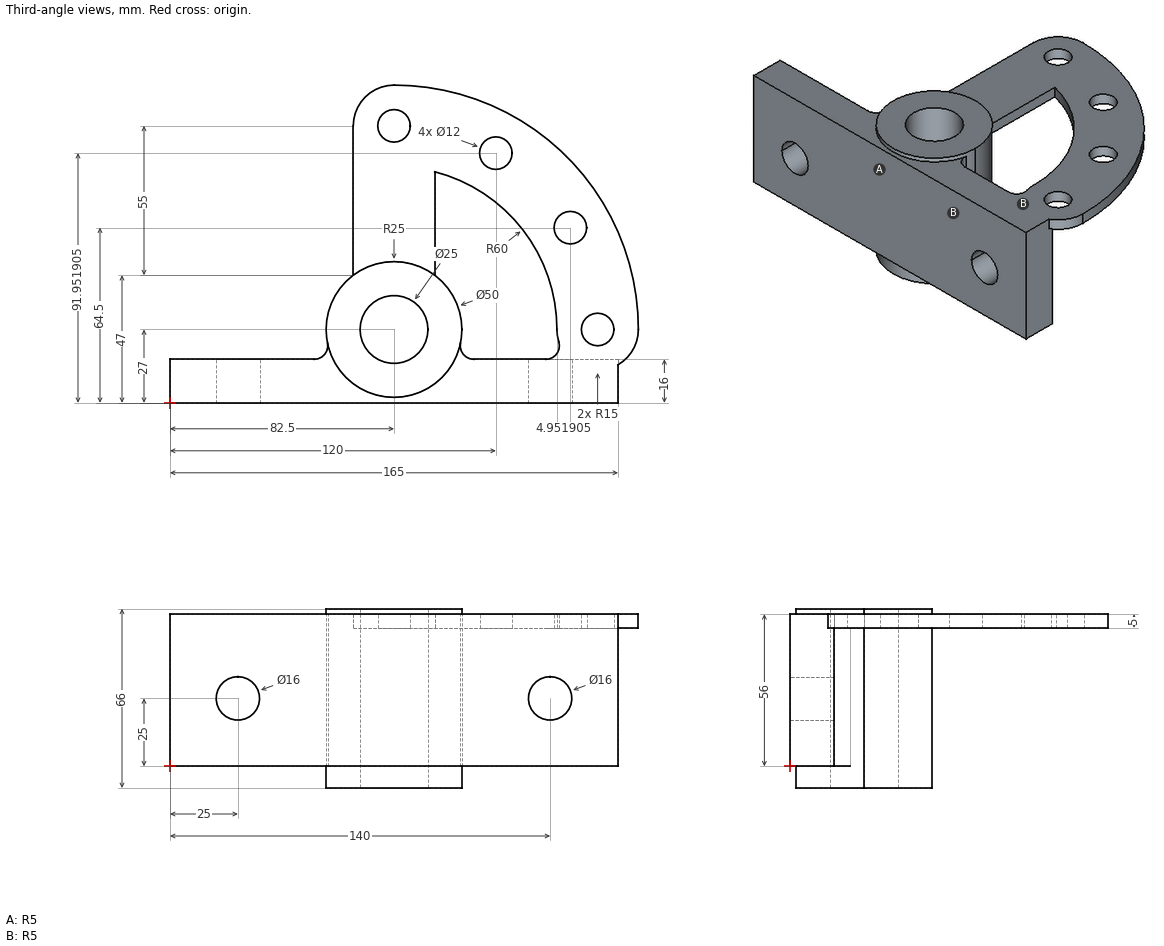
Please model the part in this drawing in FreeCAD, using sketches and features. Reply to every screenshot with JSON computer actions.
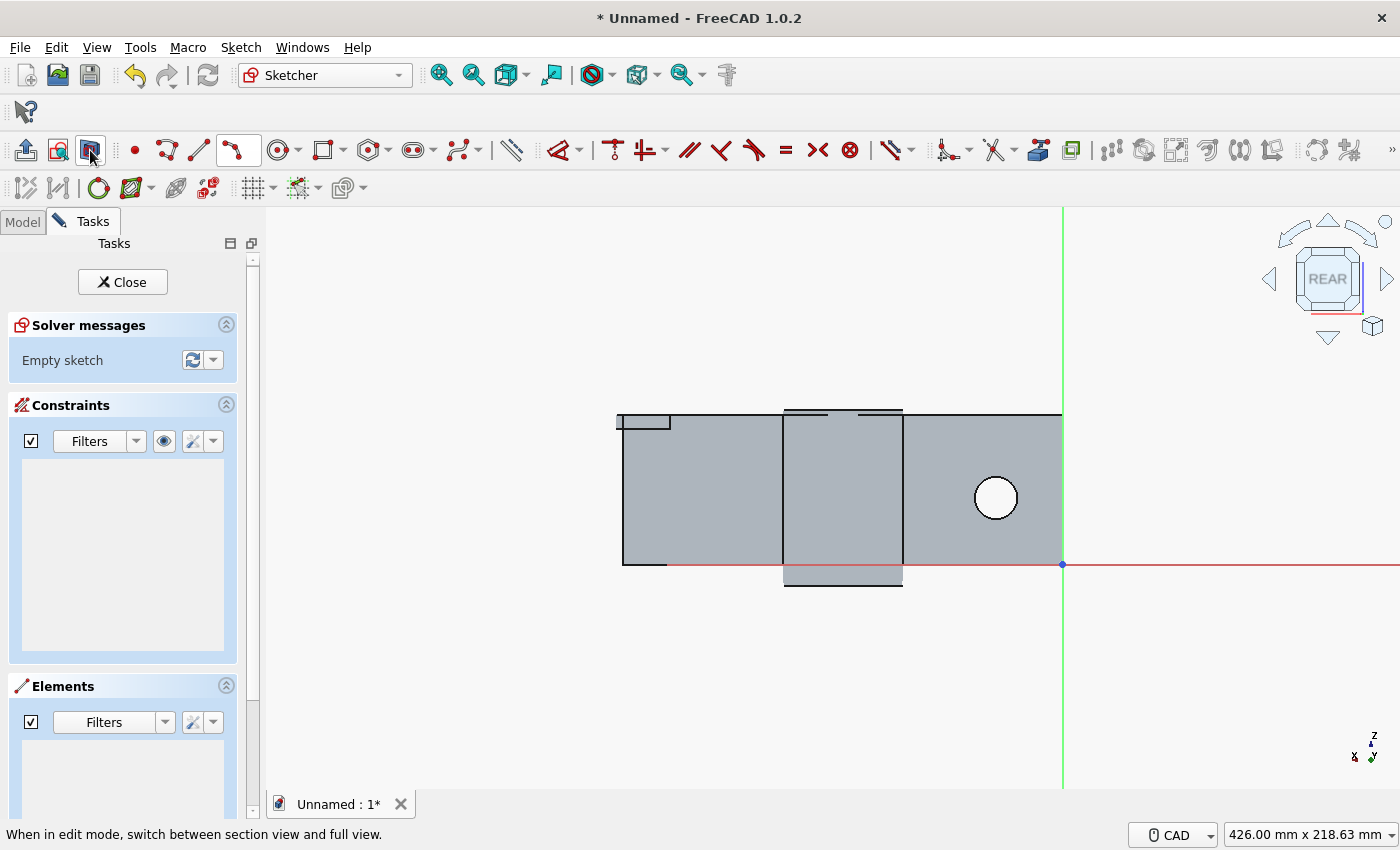
{"action": "scroll", "coordinate": [681, 498], "scroll_direction": "up", "scroll_amount": 11}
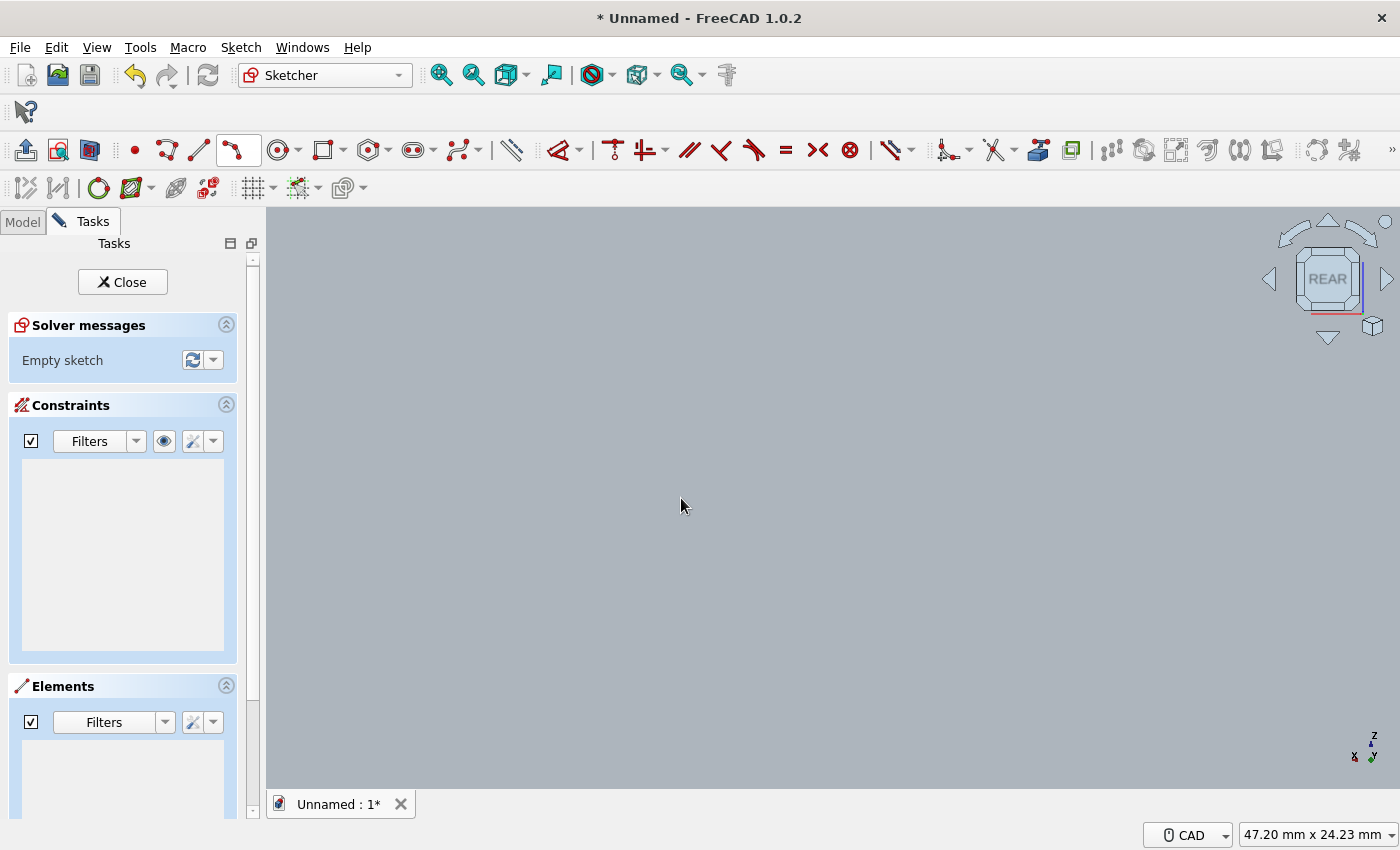
{"action": "left_click", "coordinate": [278, 150]}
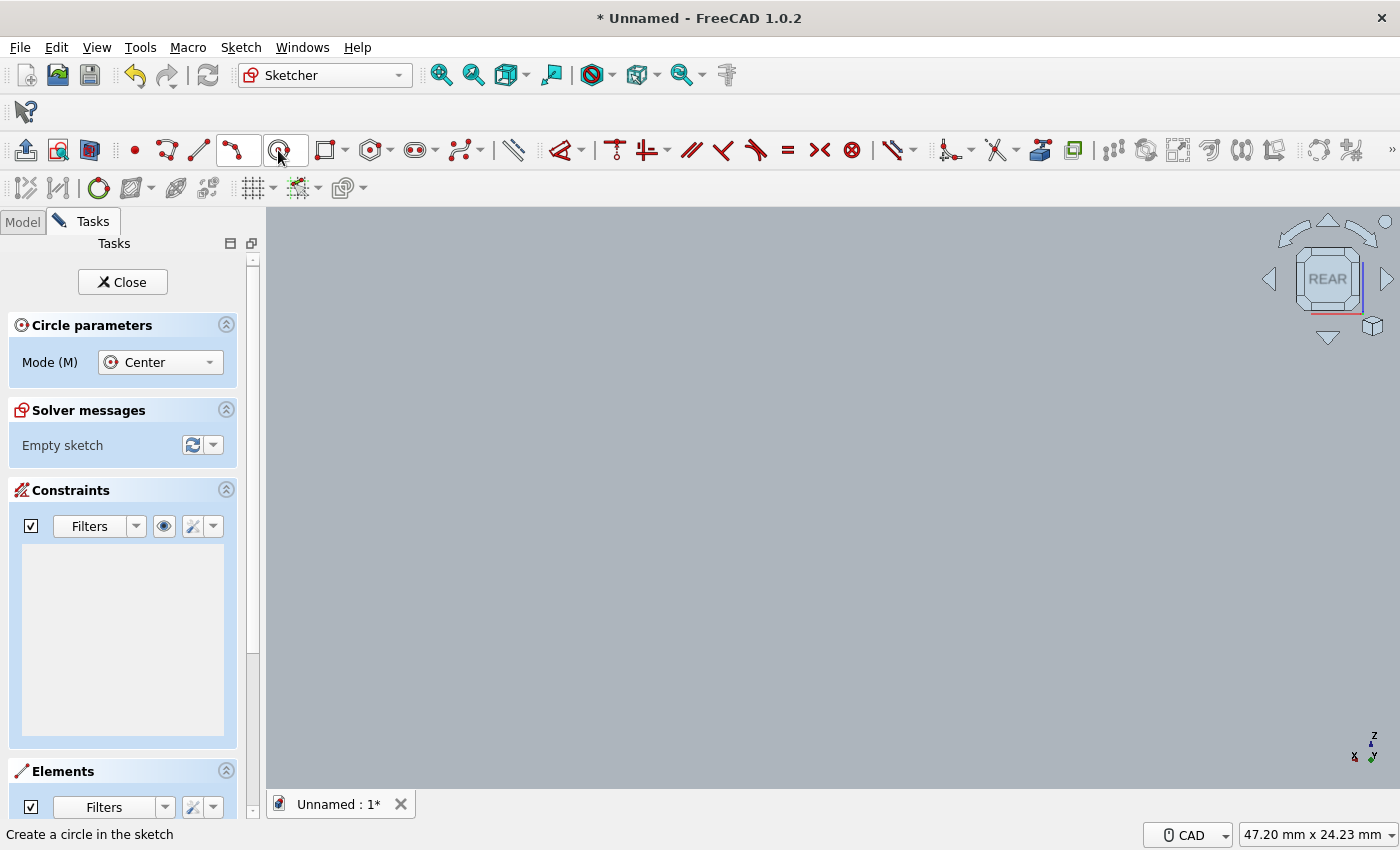
{"action": "left_click", "coordinate": [759, 494]}
{"action": "left_click", "coordinate": [894, 358]}
{"action": "key", "text": "Escape"}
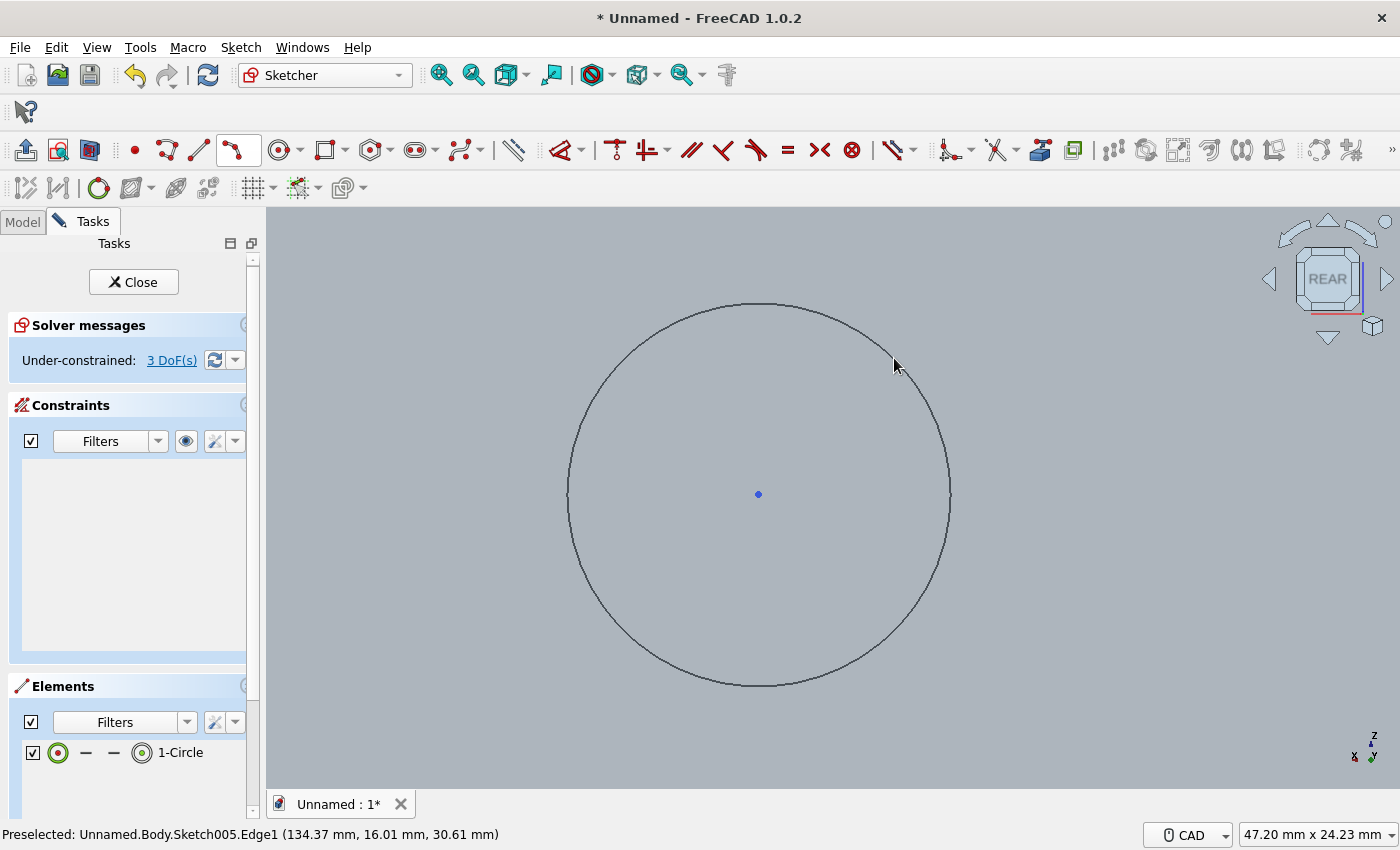
{"action": "left_click", "coordinate": [560, 150]}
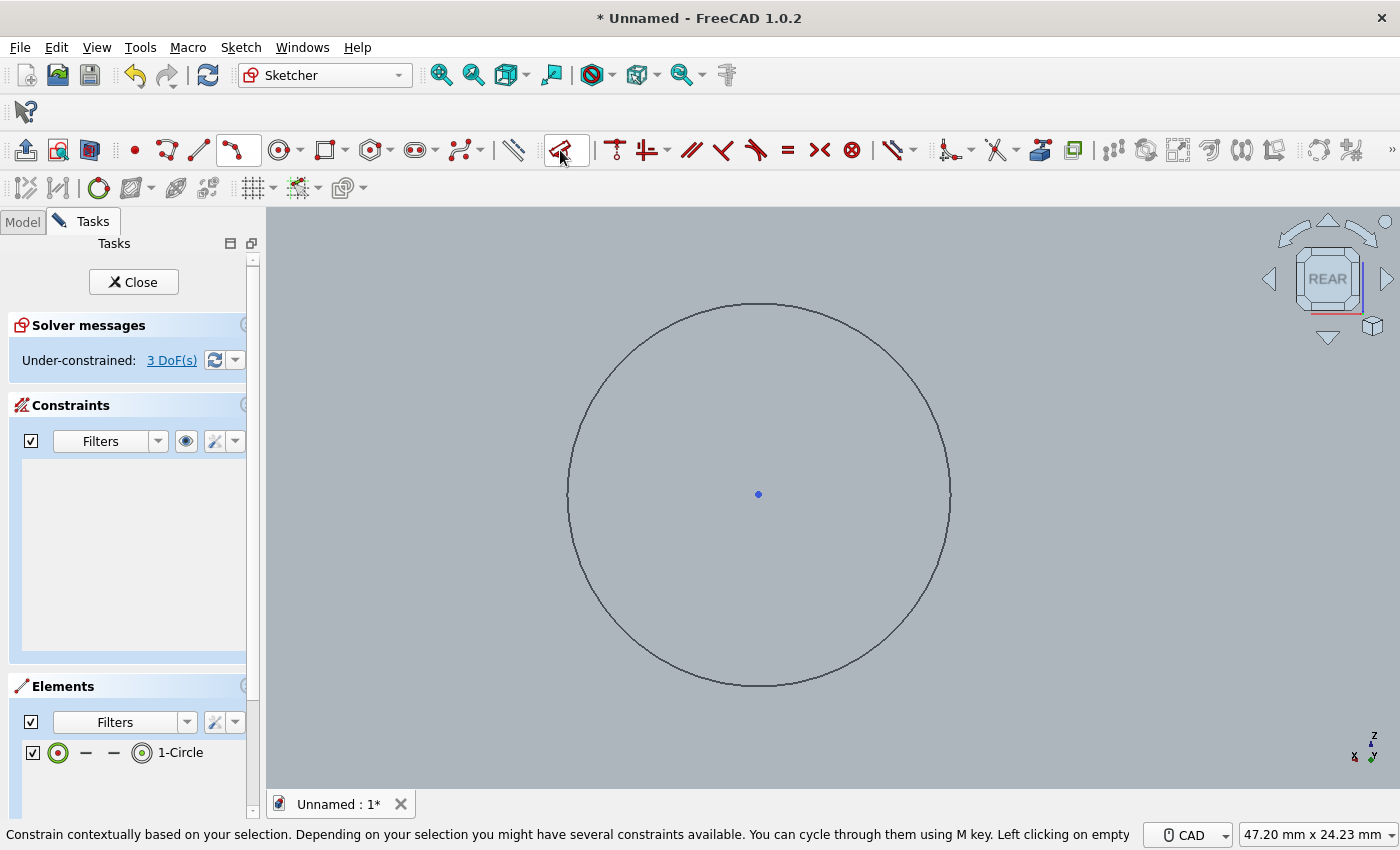
{"action": "left_click", "coordinate": [894, 359]}
{"action": "left_click", "coordinate": [917, 336]}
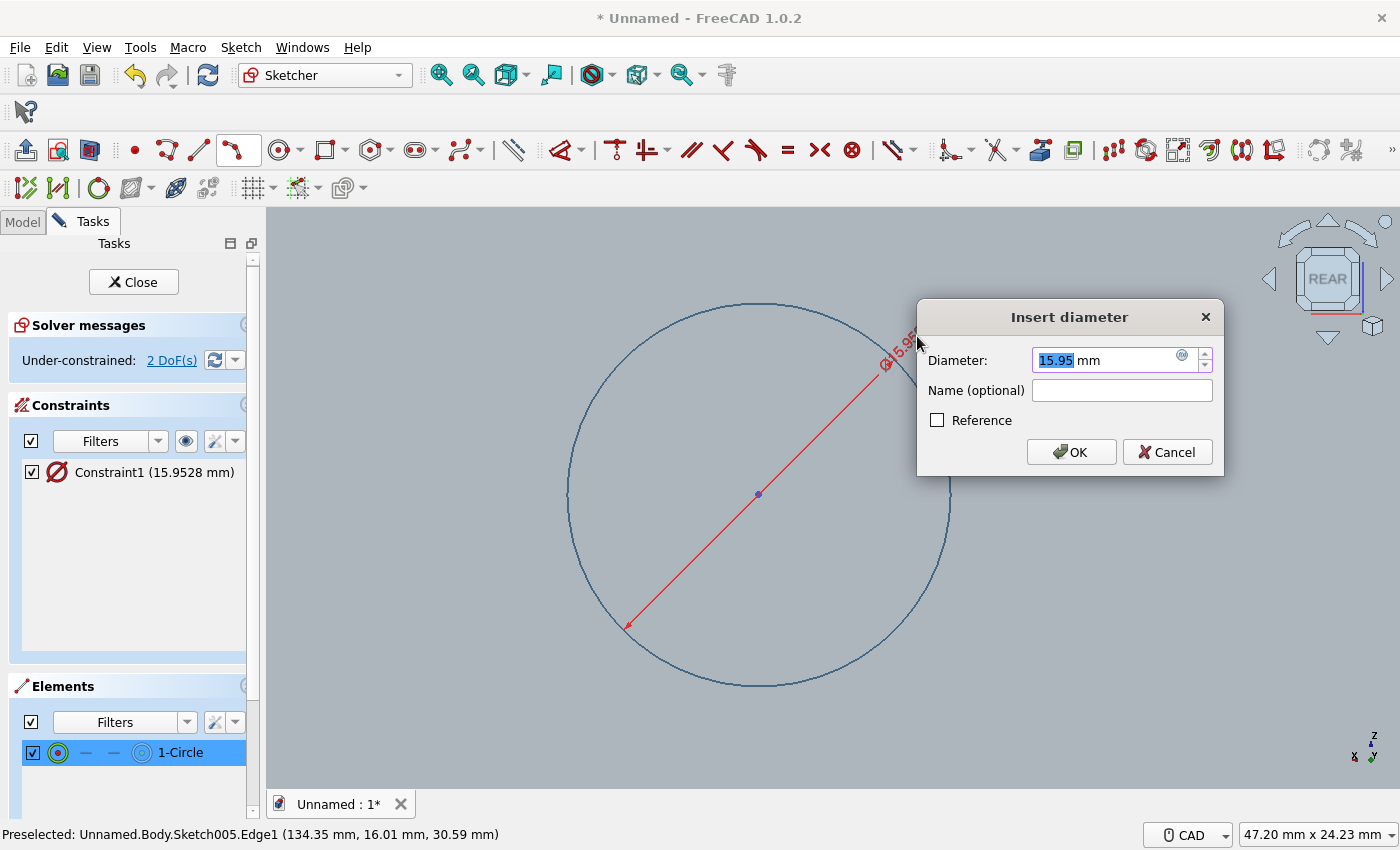
{"action": "type", "text": "16"}
{"action": "key", "text": "Return"}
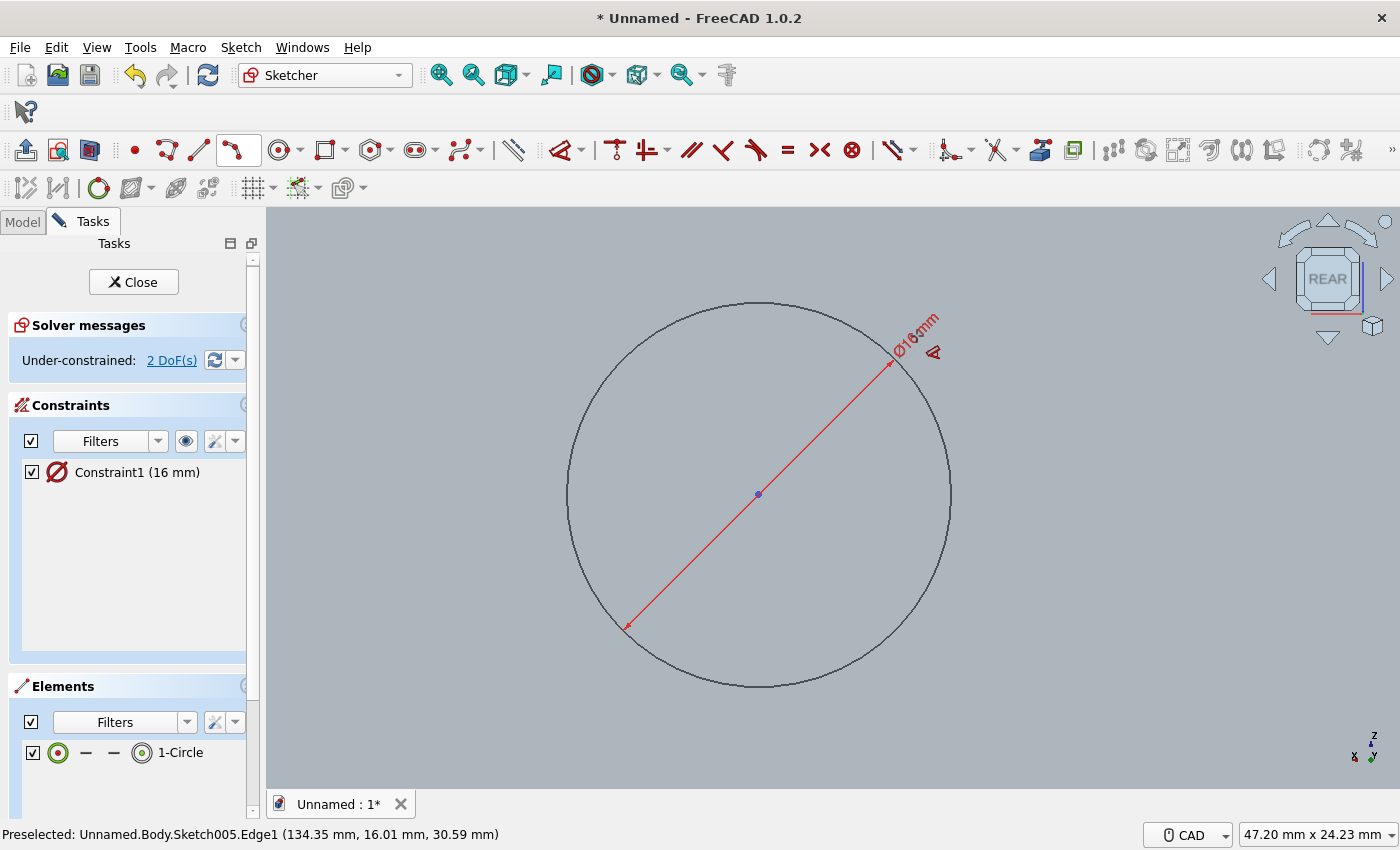
{"action": "left_click", "coordinate": [759, 495]}
{"action": "left_click", "coordinate": [725, 628]}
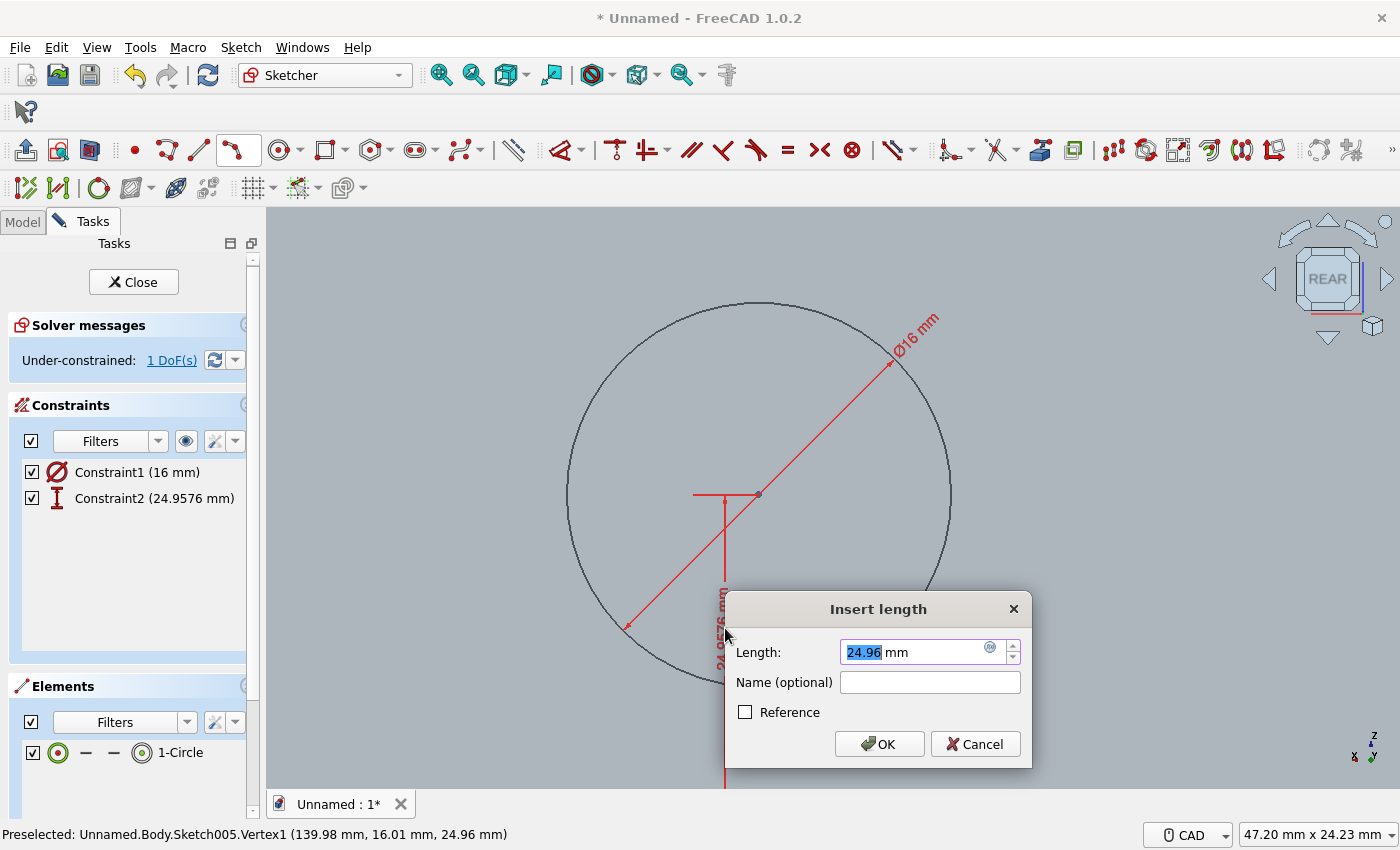
{"action": "type", "text": "25"}
{"action": "key", "text": "Return"}